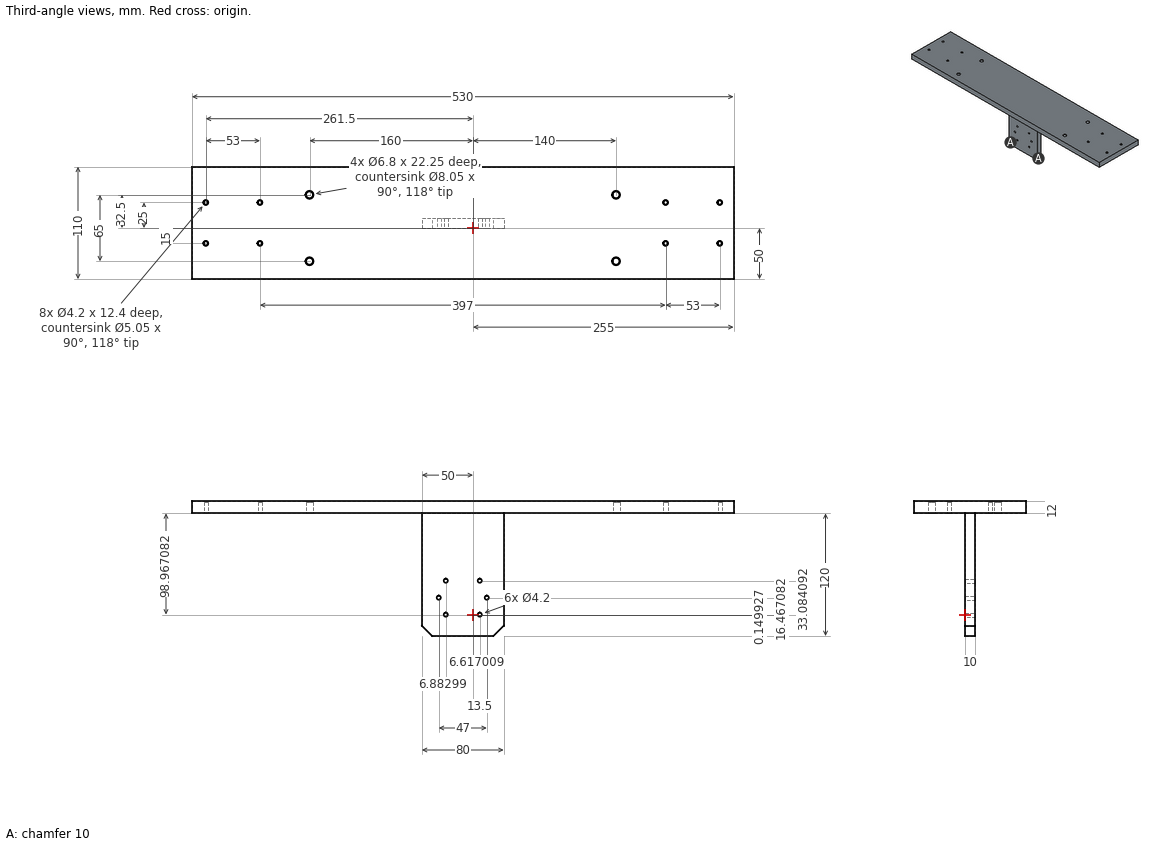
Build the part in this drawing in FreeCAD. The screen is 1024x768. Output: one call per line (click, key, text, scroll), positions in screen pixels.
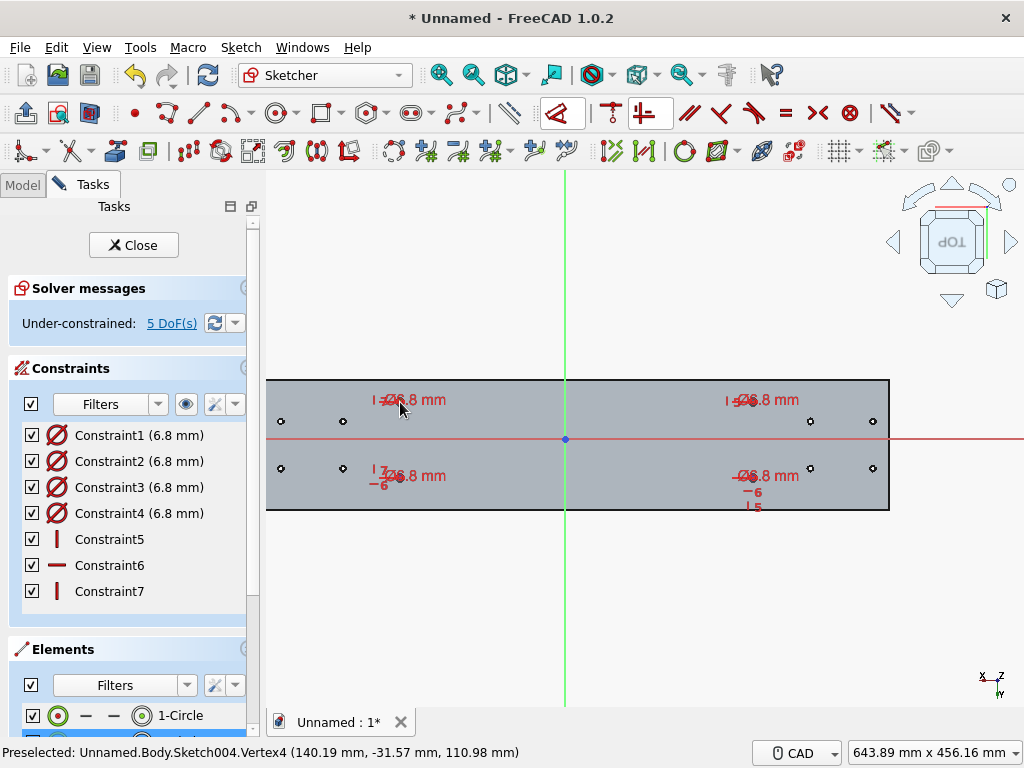
key(h)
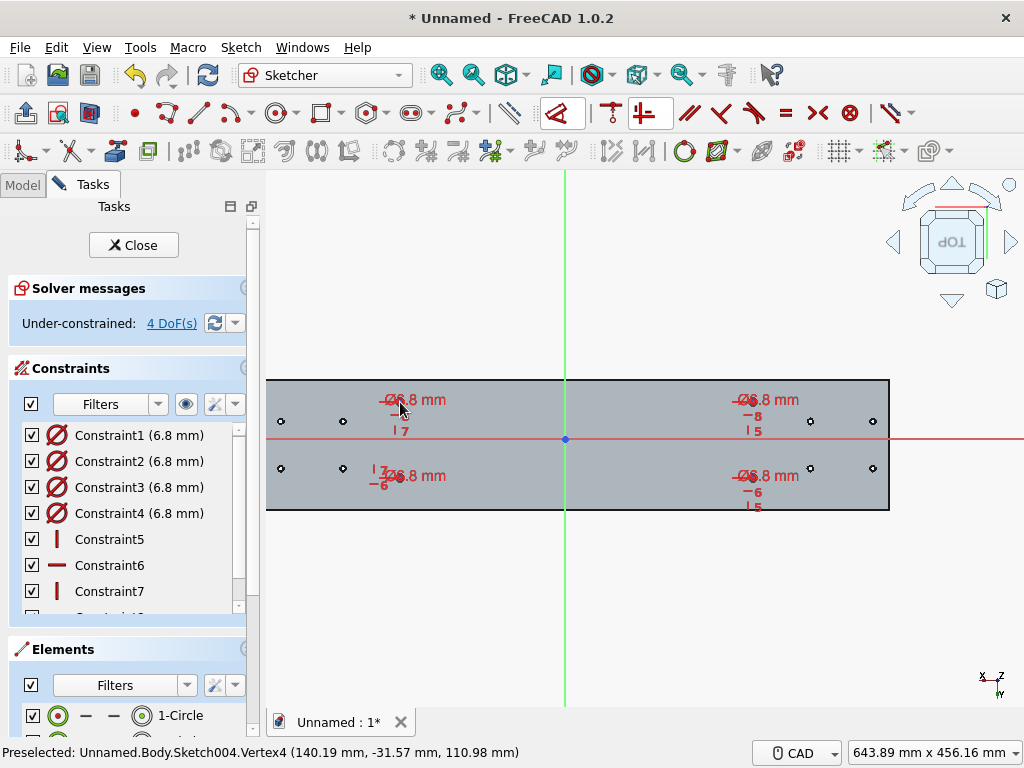
click(753, 478)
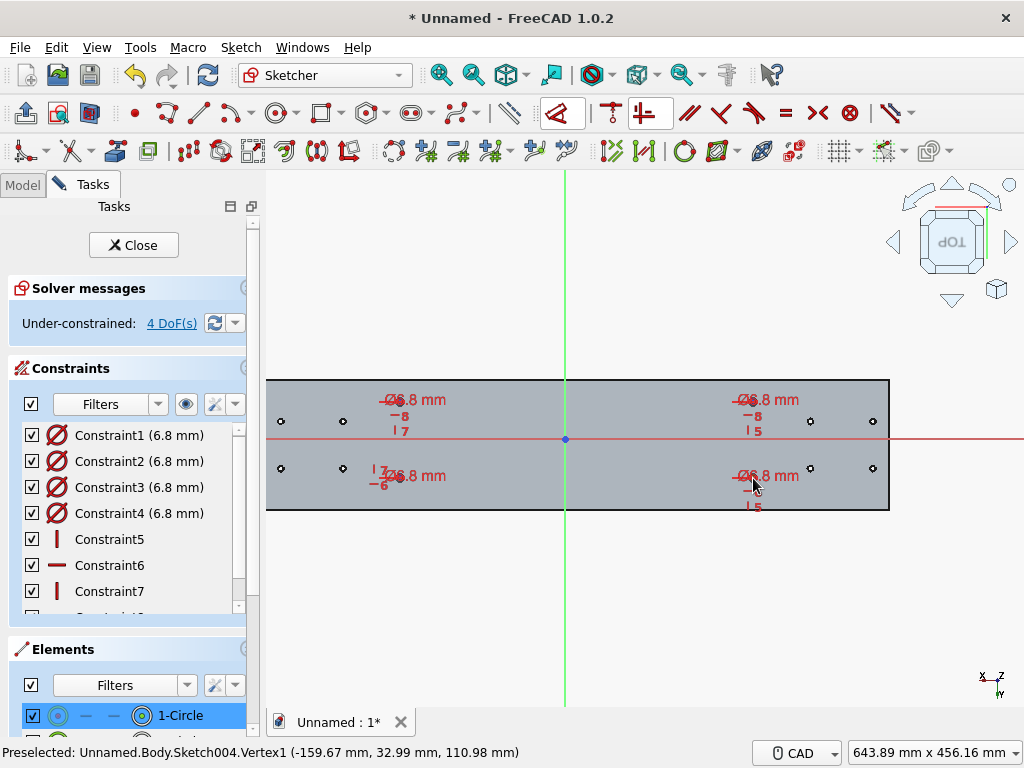
key(l)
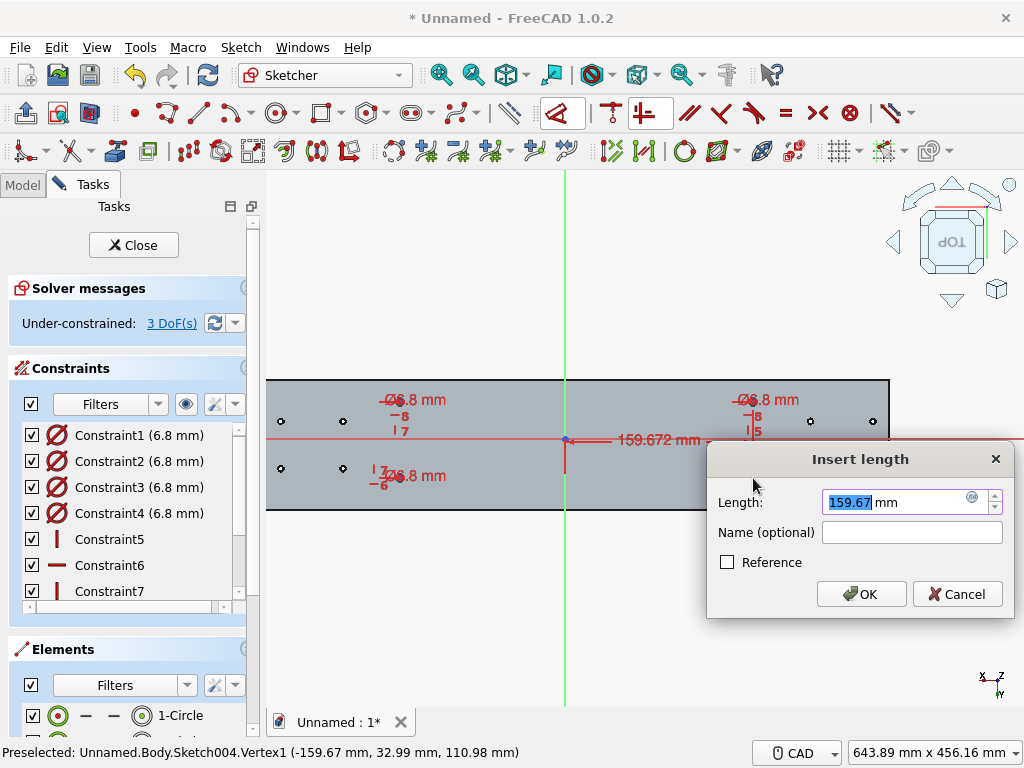
text(160)
key(Return)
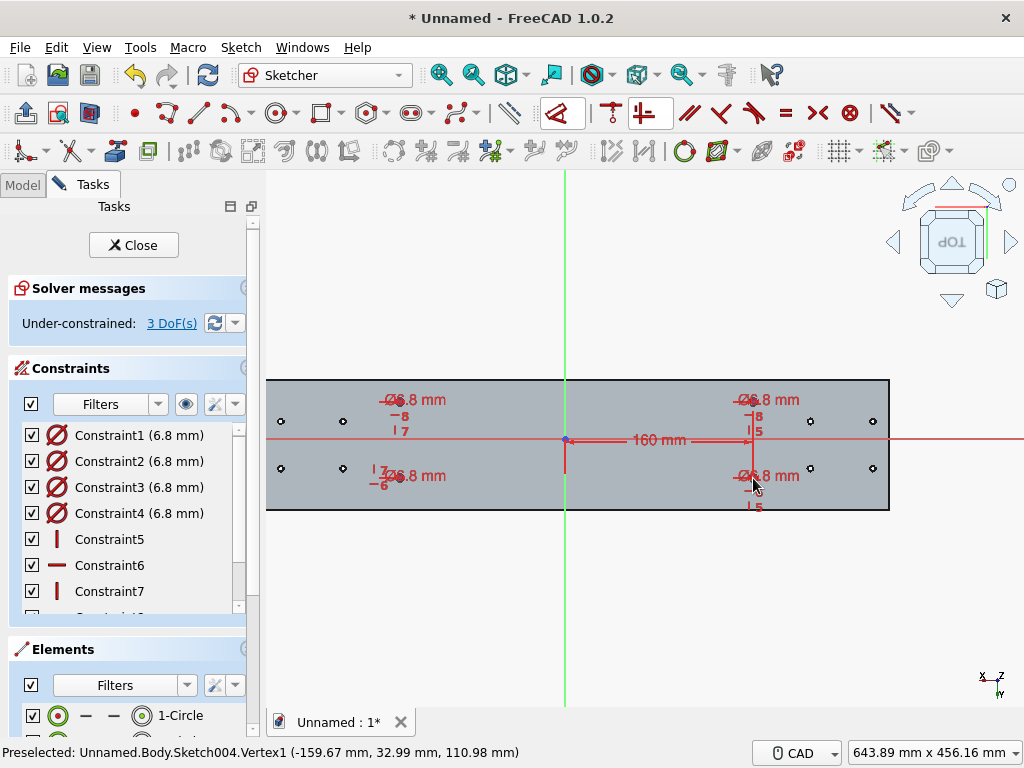
click(400, 478)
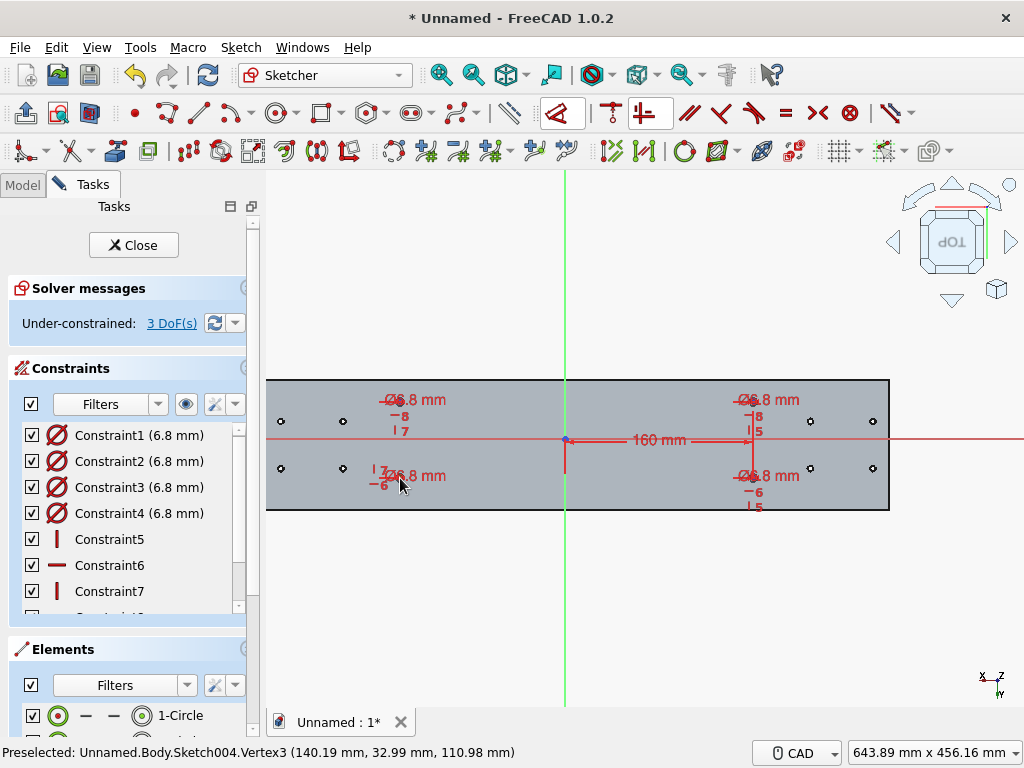
key(l)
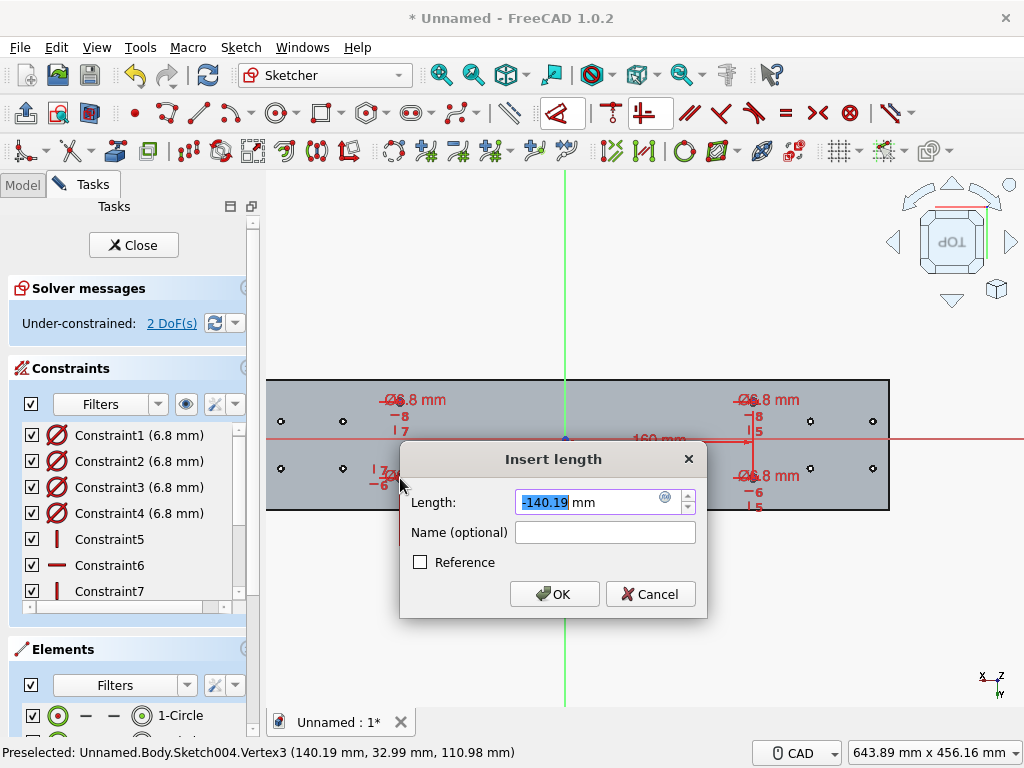
text(-140)
key(Return)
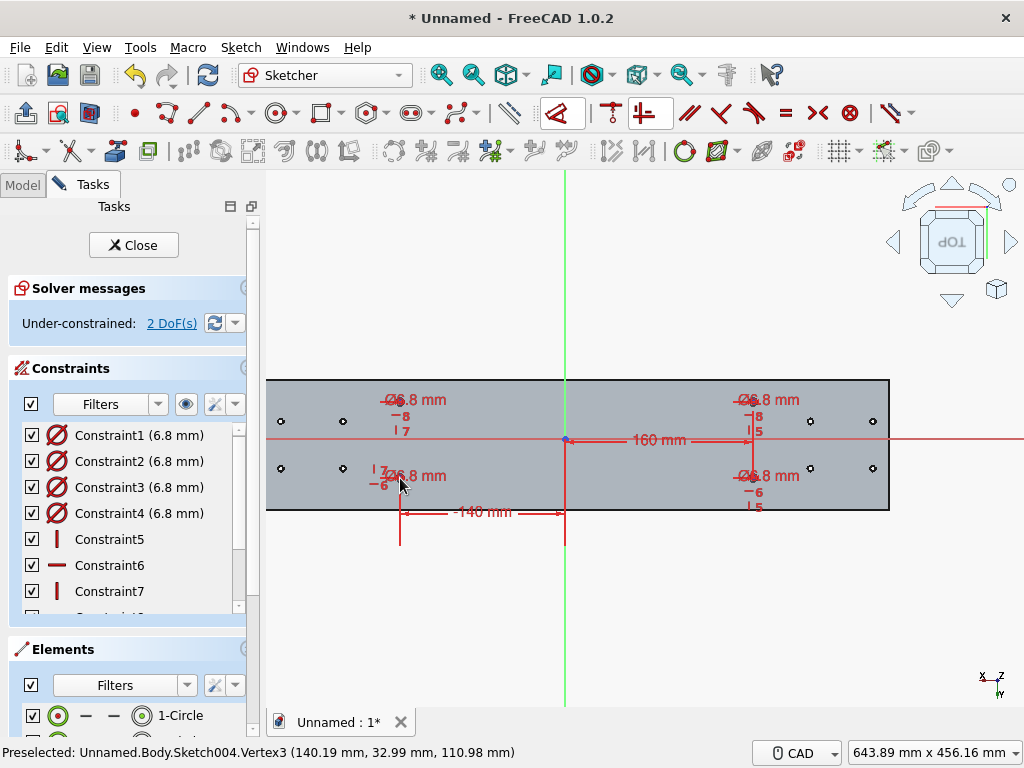
click(753, 478)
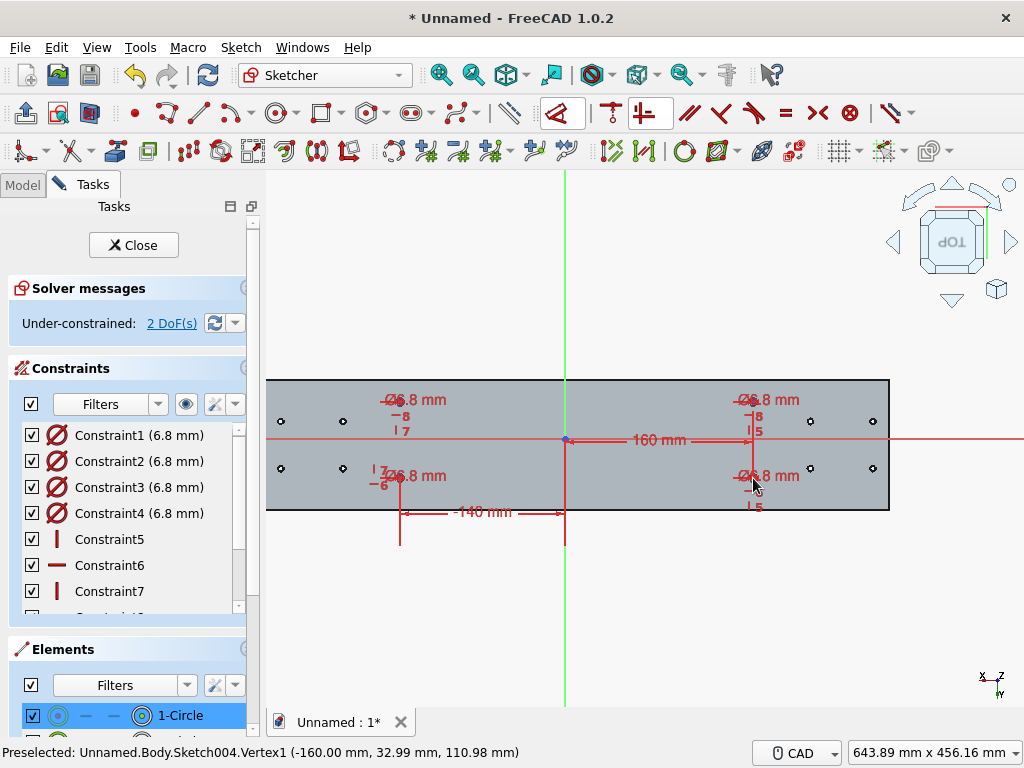
click(753, 402)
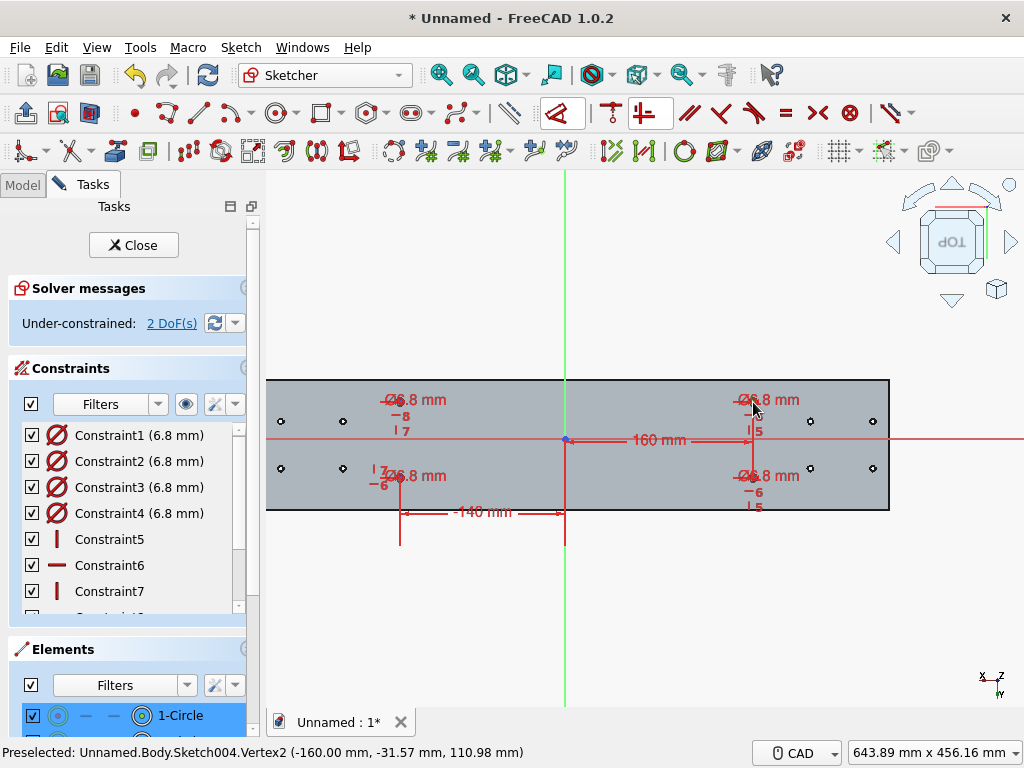
click(580, 114)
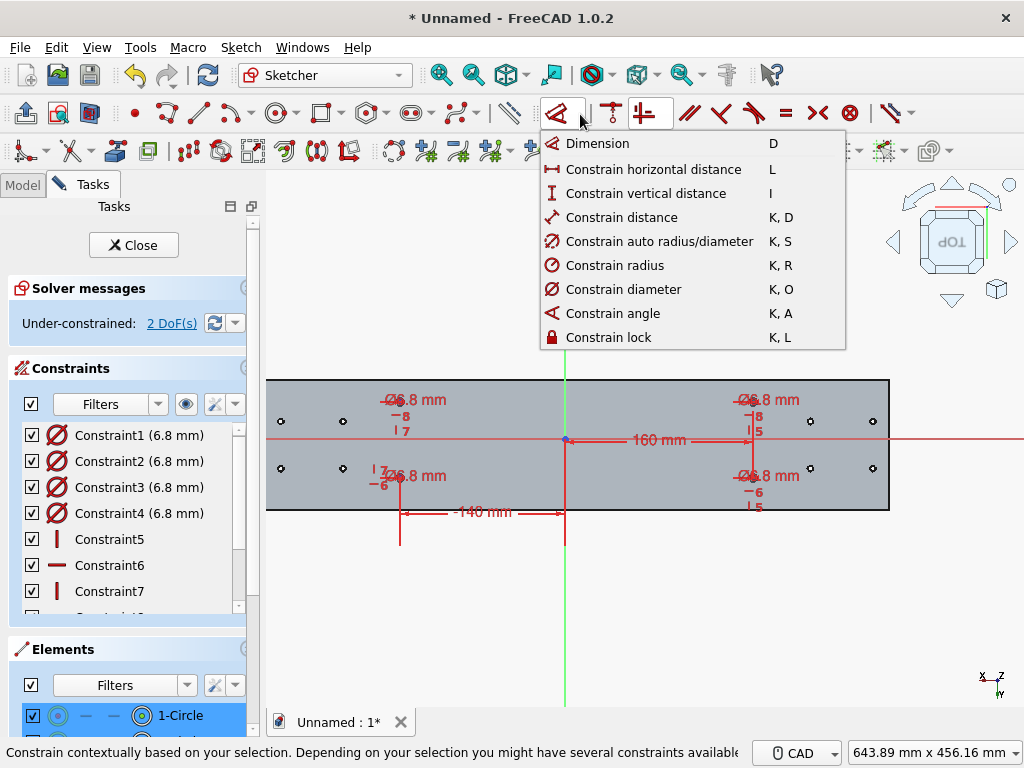
click(693, 193)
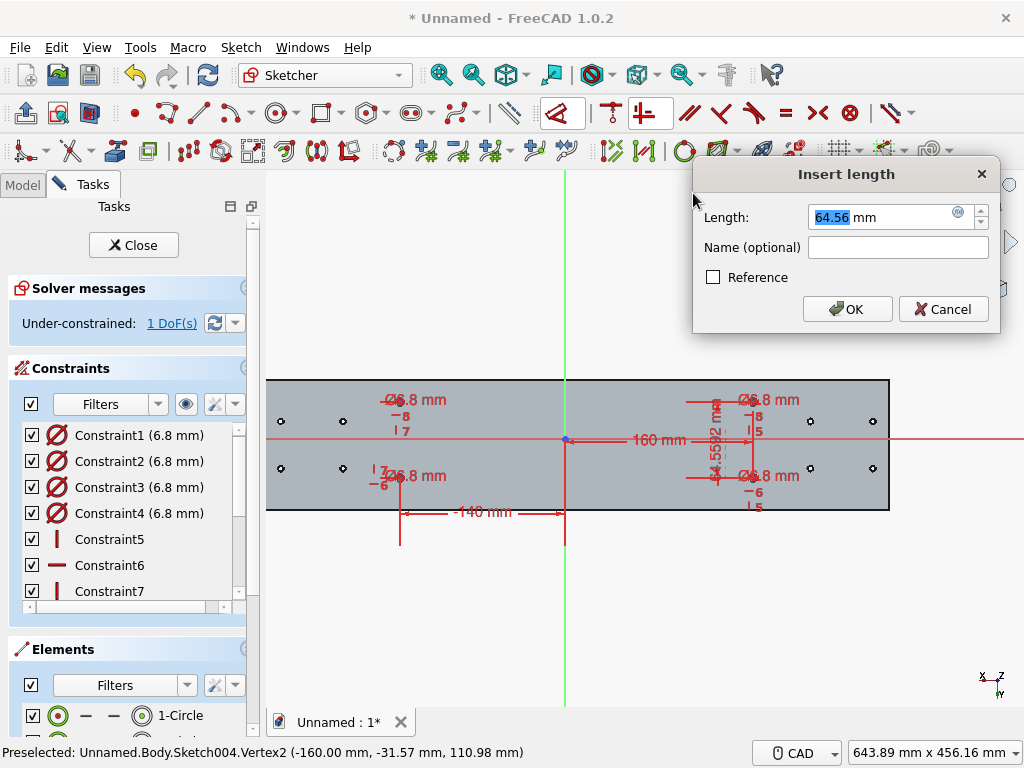
text(65)
key(Return)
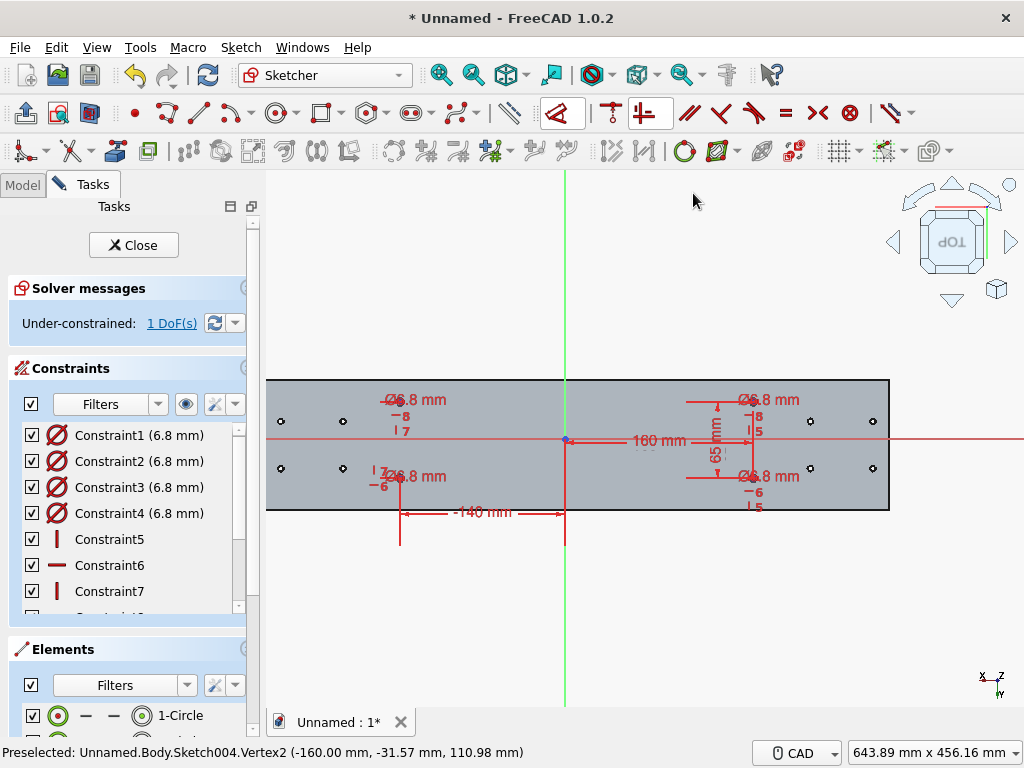
click(753, 478)